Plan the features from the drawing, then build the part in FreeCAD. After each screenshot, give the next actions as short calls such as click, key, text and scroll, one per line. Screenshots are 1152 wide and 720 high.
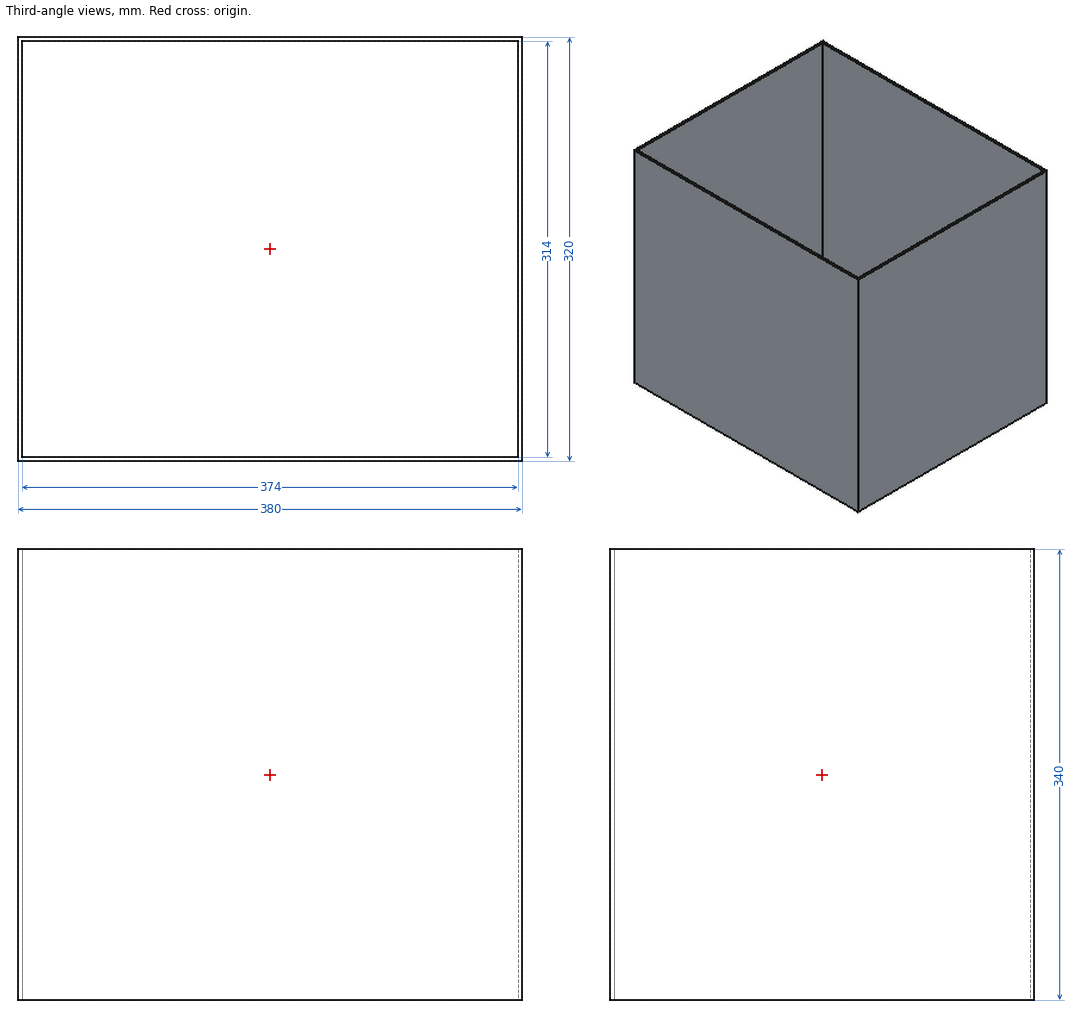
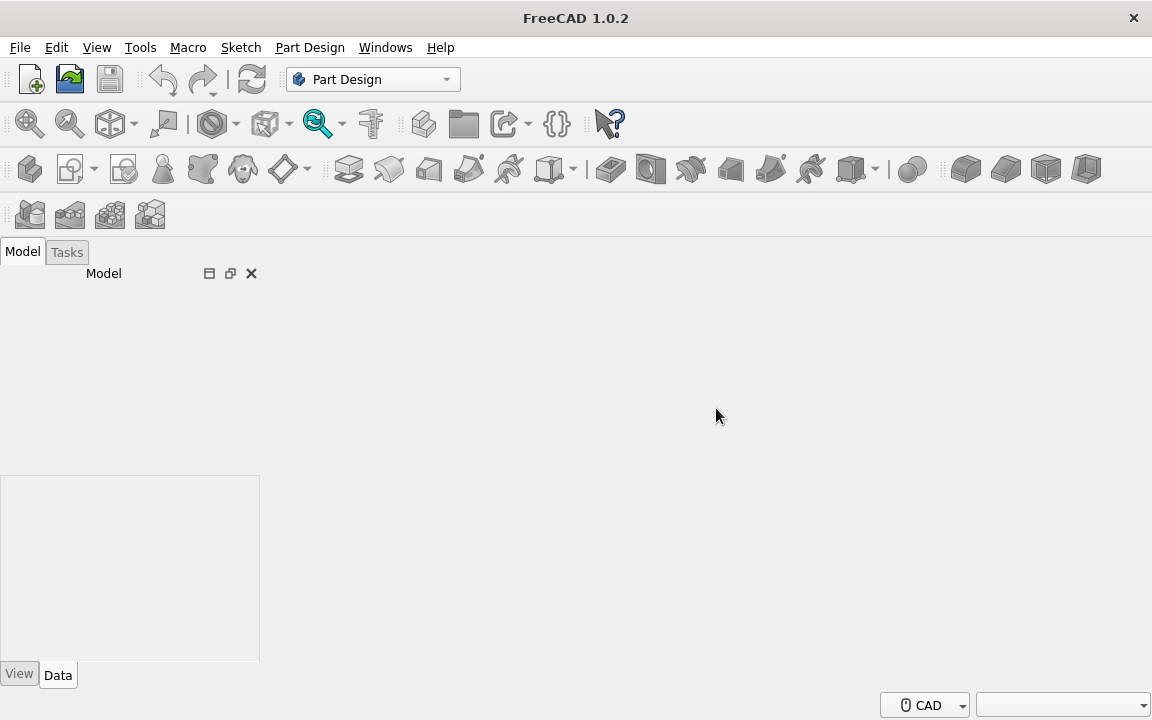
key(ctrl+n)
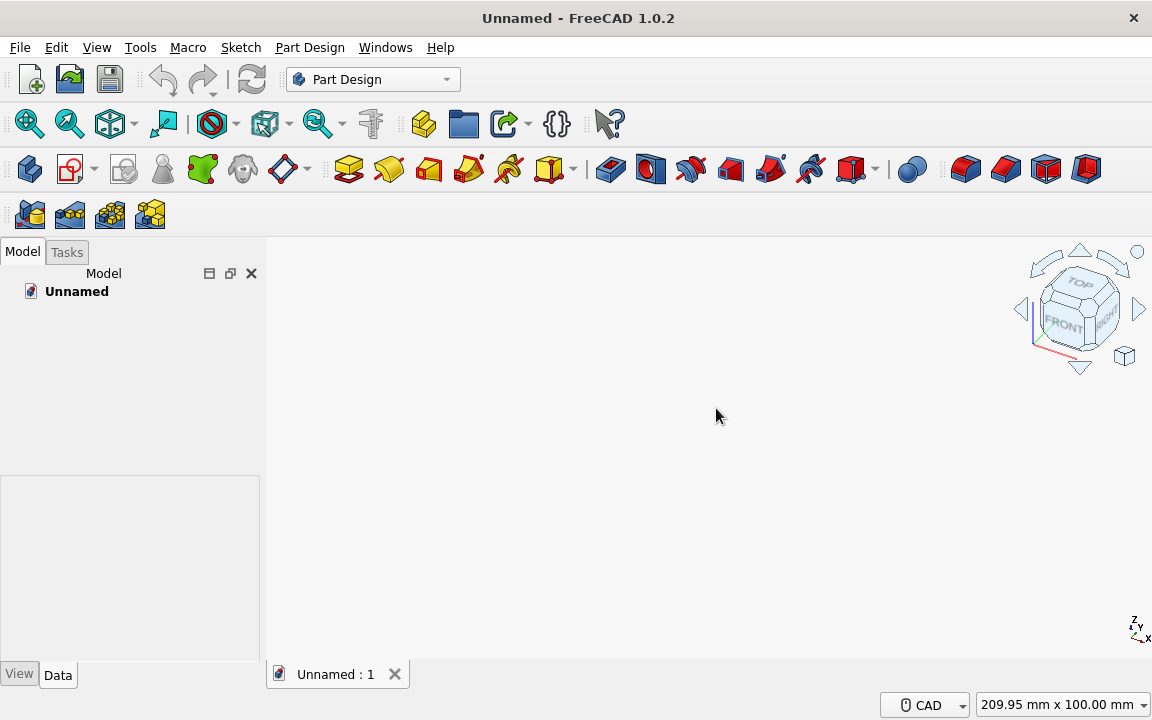
click(70, 170)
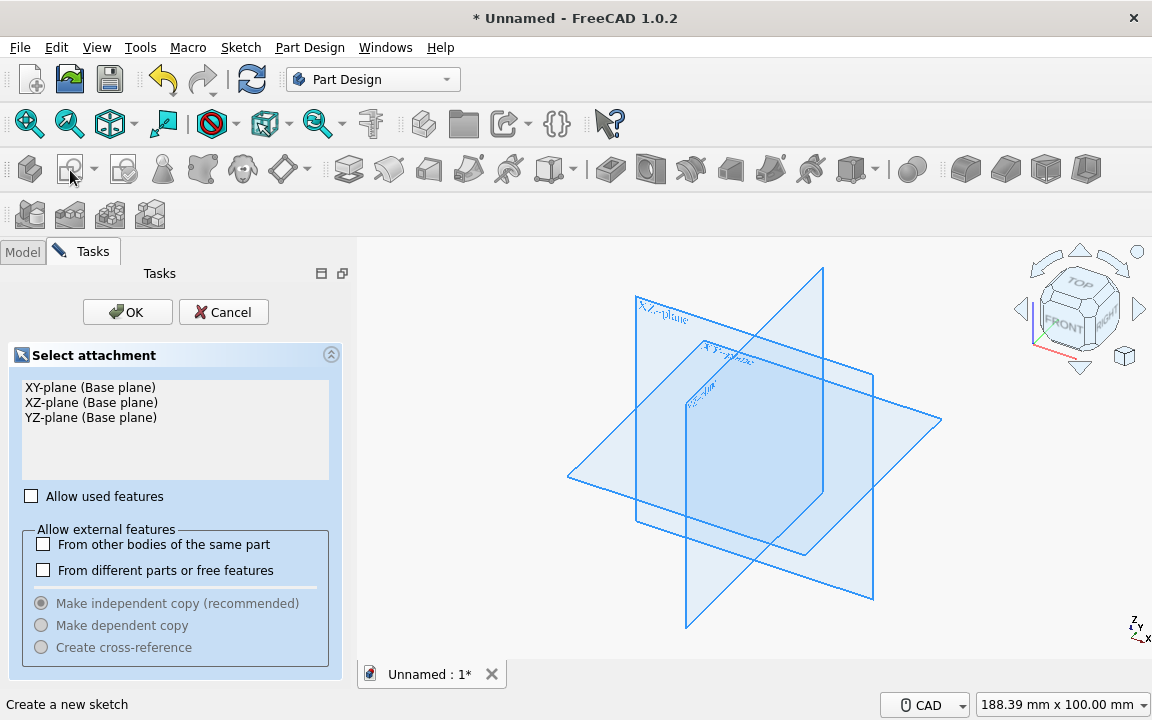
click(82, 388)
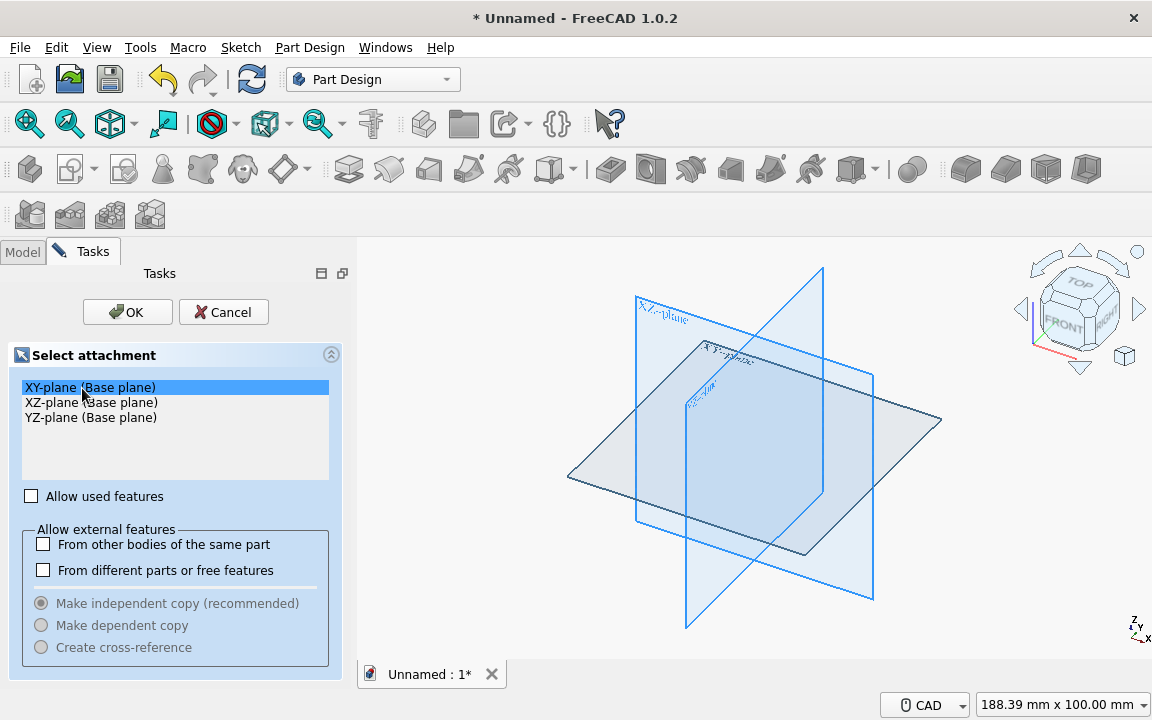
click(128, 312)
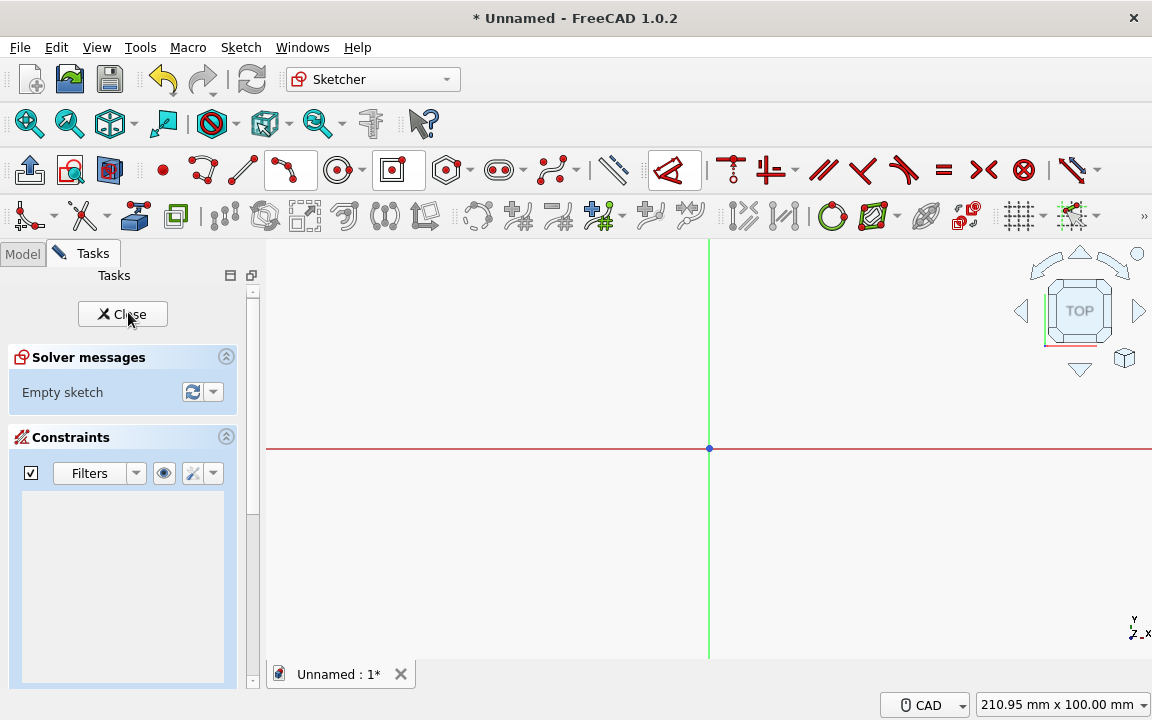
scroll(623, 449, down, 8)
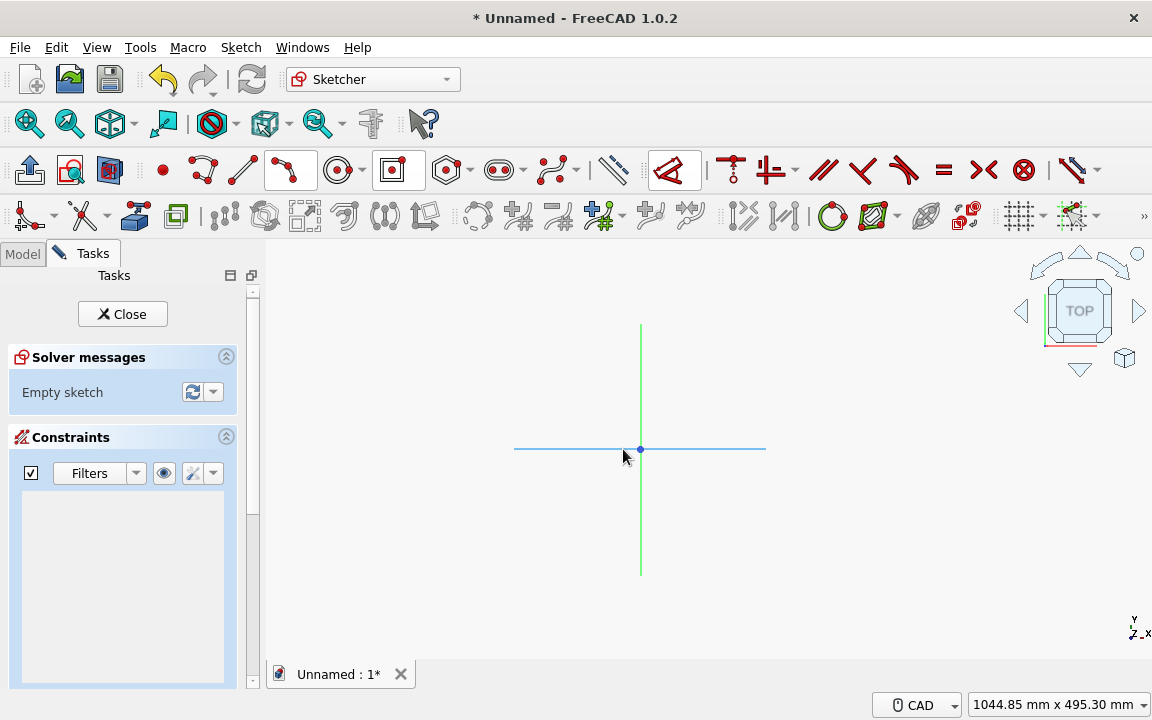
click(392, 170)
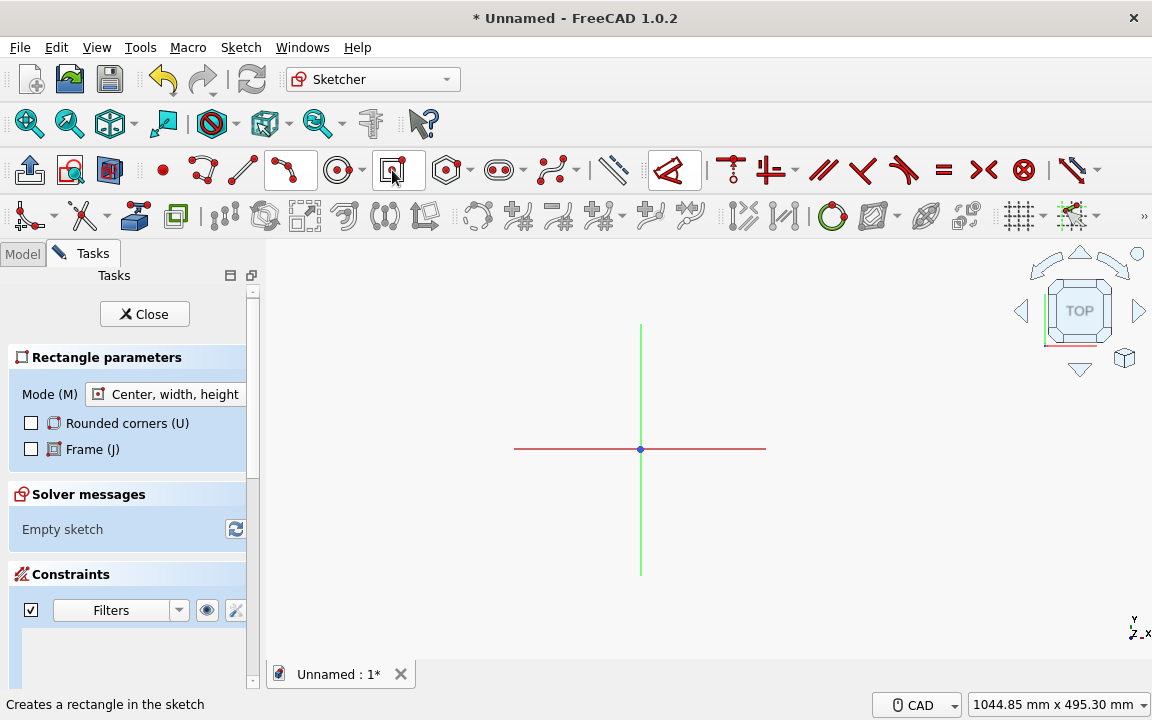
click(641, 449)
move(802, 314)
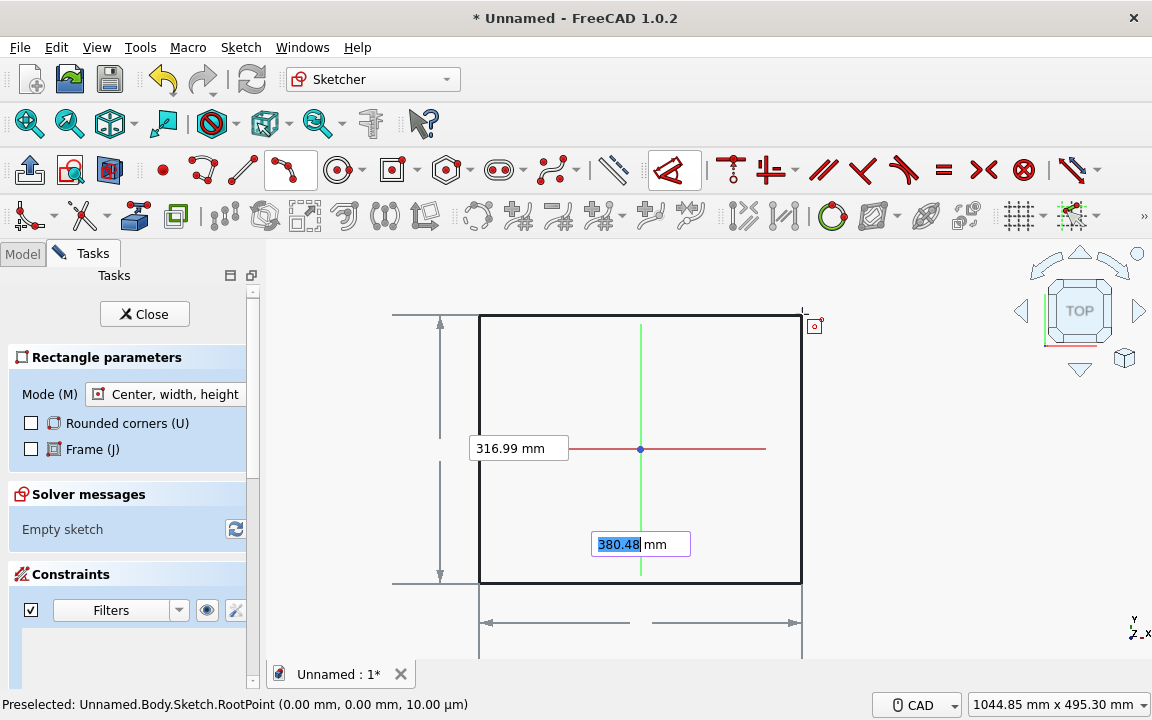
text(380)
key(Tab)
text(320)
key(Return)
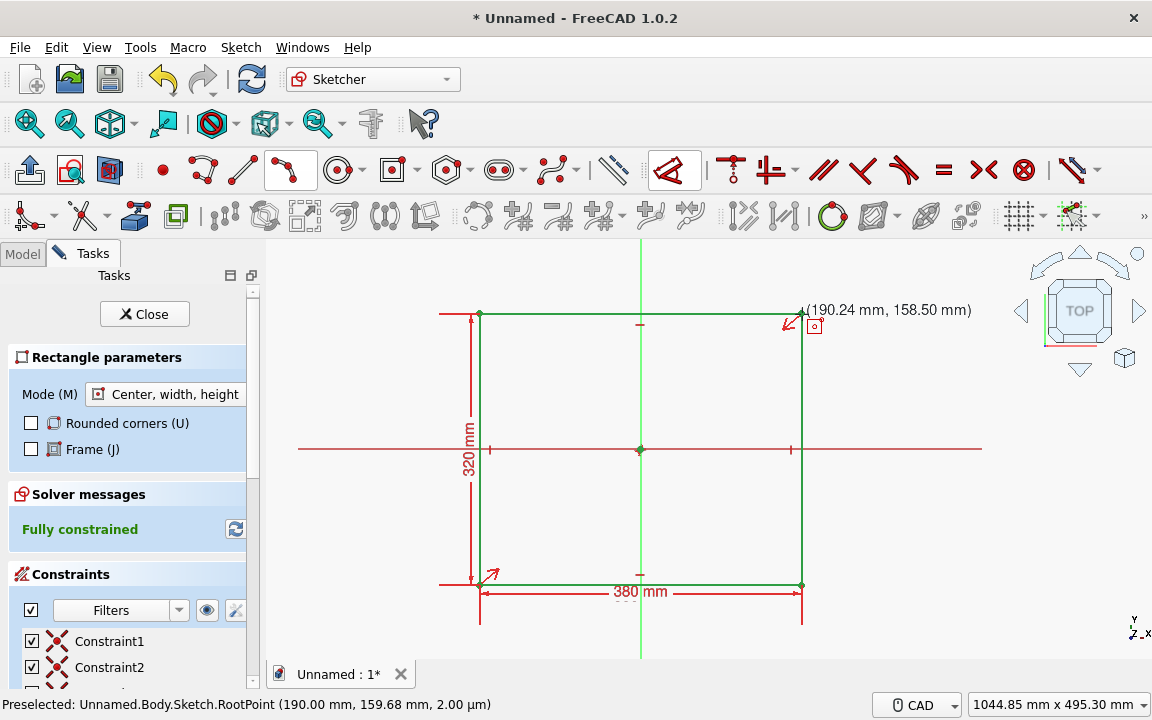
click(641, 449)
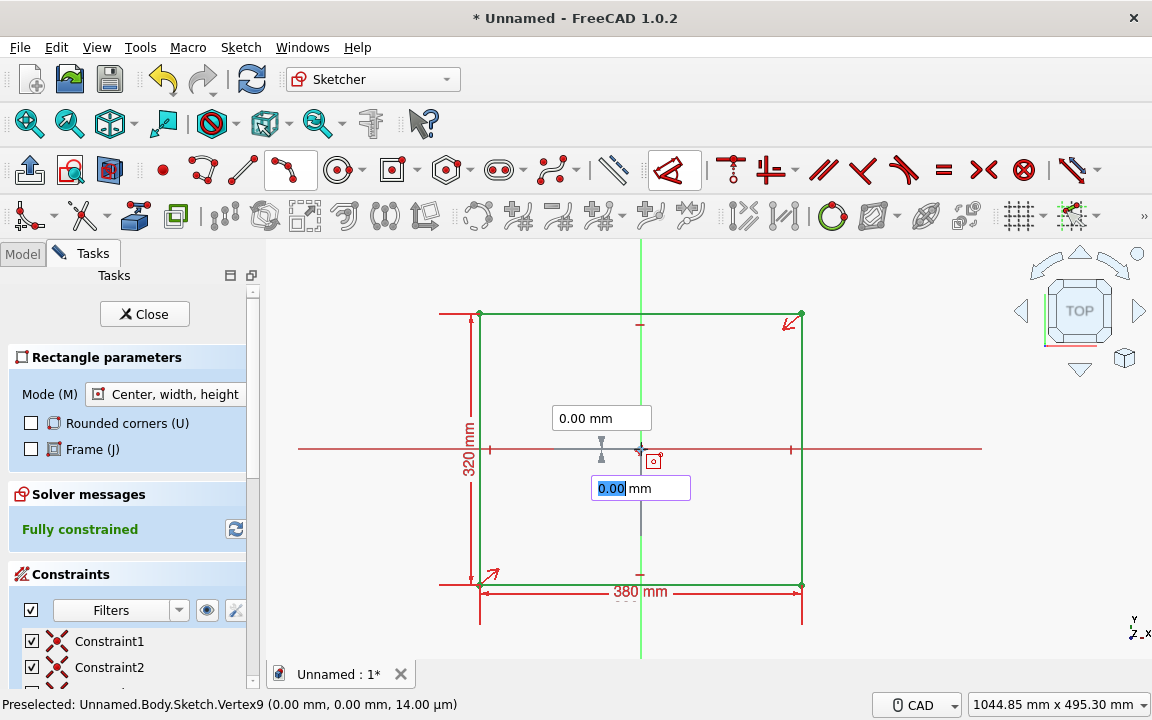
scroll(799, 316, up, 10)
move(797, 317)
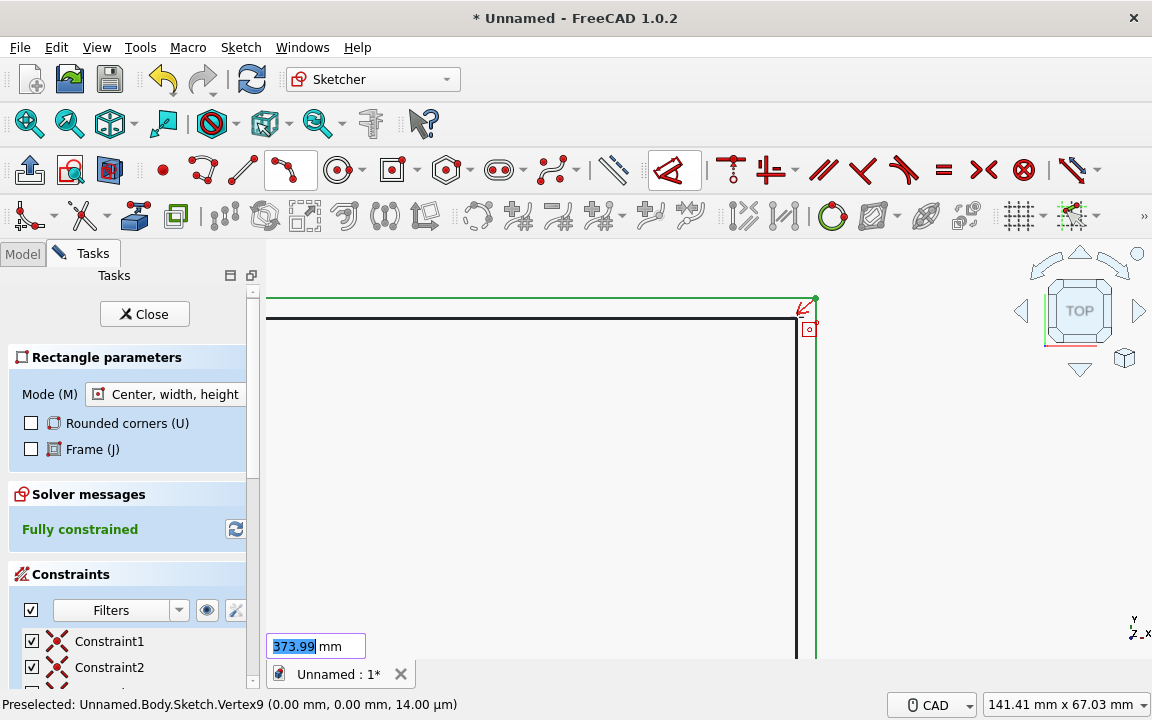
text(374)
key(Tab)
text(314)
key(Return)
key(Escape)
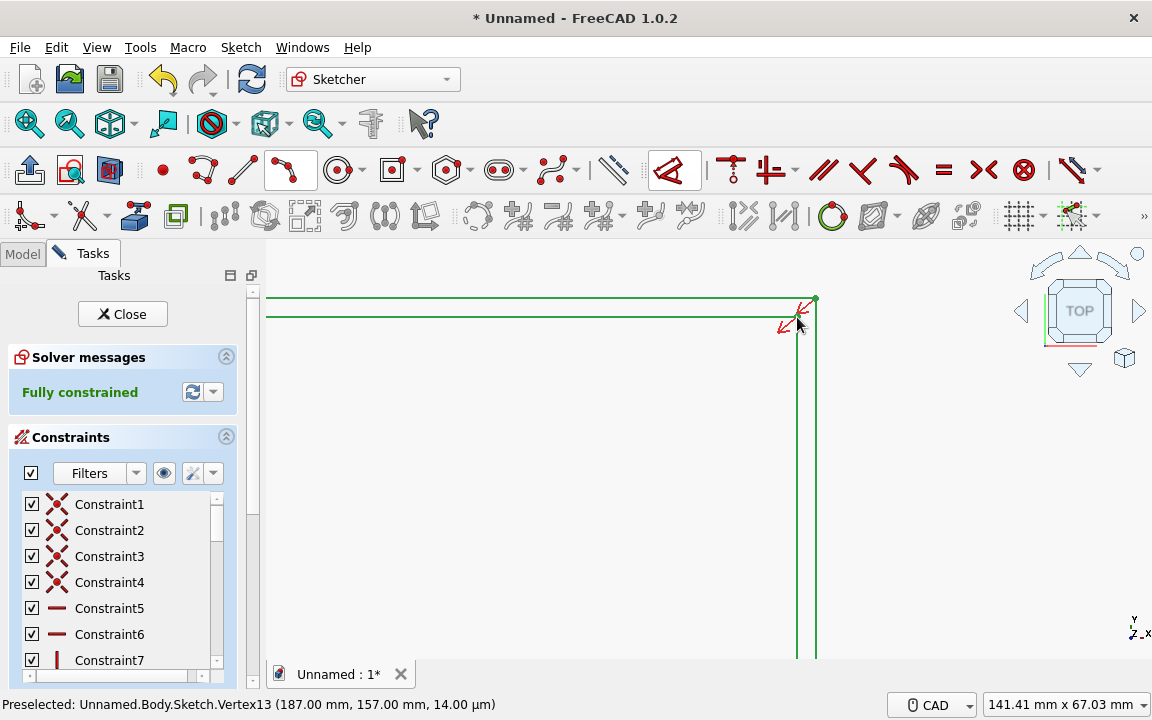
click(123, 314)